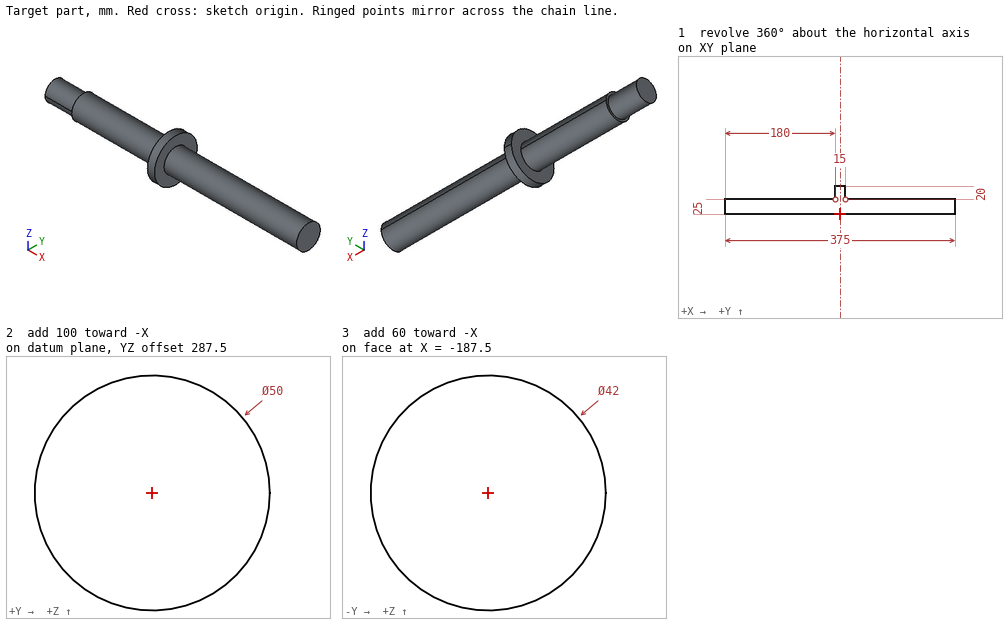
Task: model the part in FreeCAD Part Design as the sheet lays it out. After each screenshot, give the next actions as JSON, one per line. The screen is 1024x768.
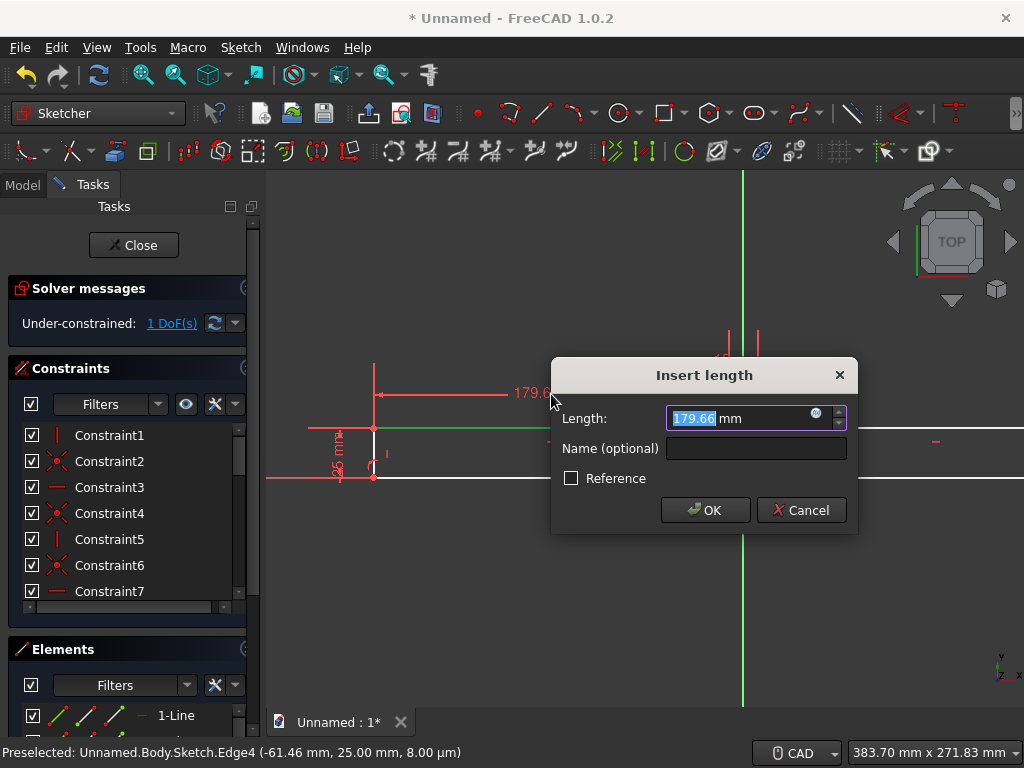
{"action": "type", "text": "180"}
{"action": "key", "text": "Return"}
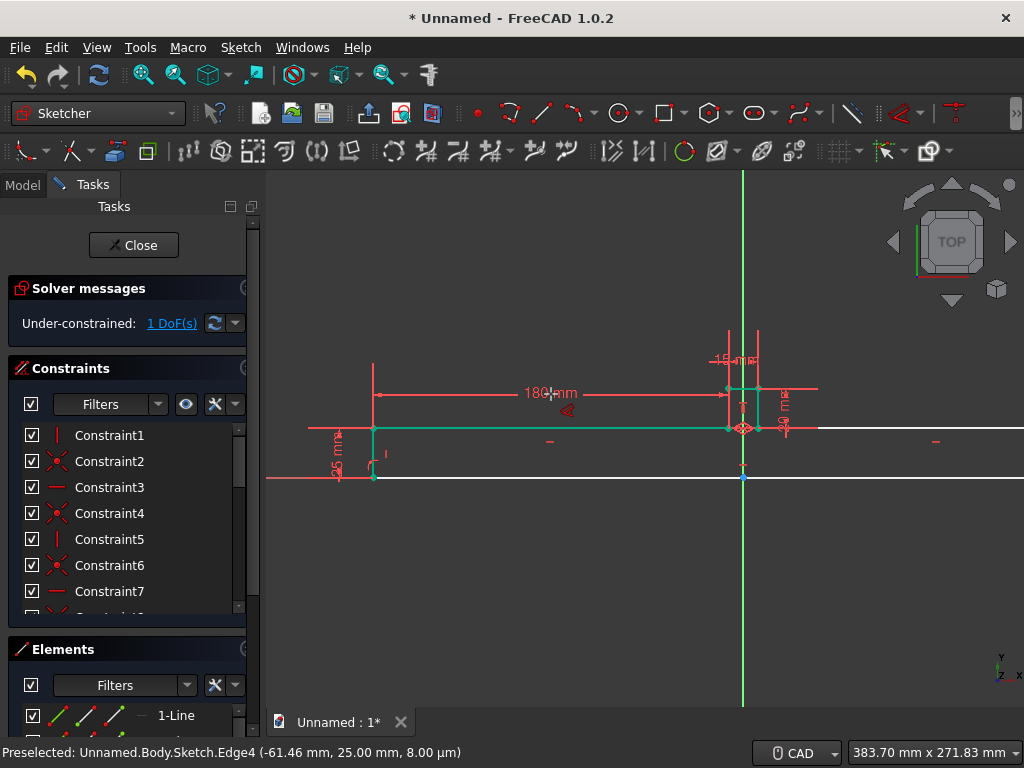
{"action": "left_click", "coordinate": [595, 478]}
{"action": "left_click", "coordinate": [616, 512]}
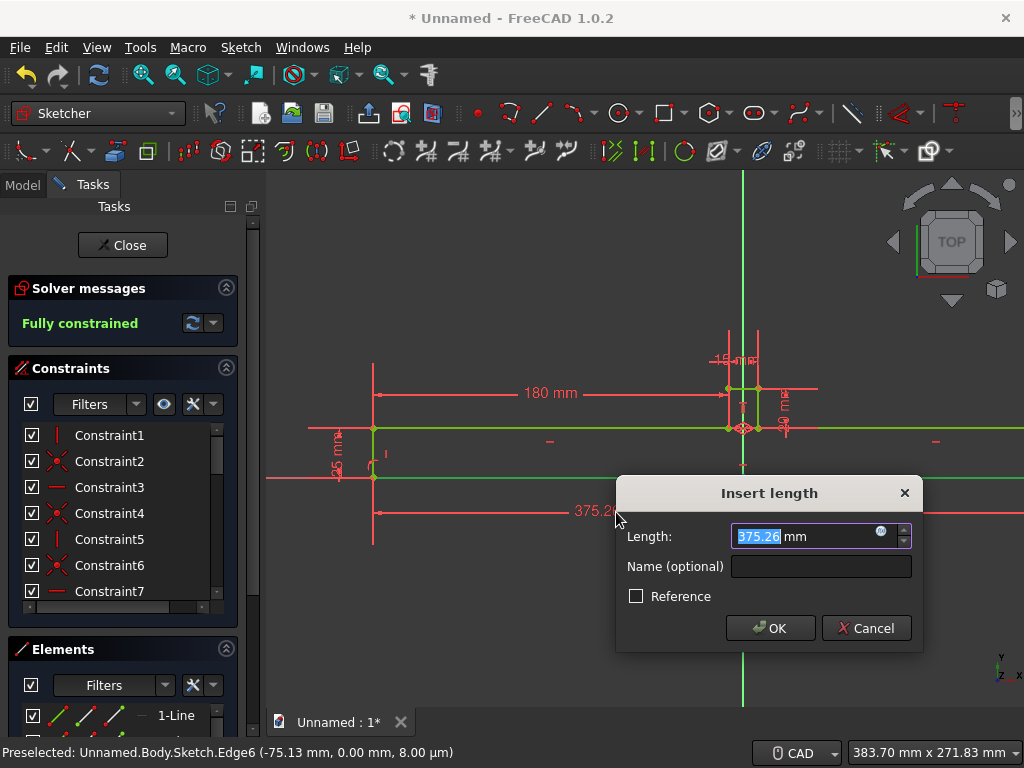
{"action": "type", "text": "375"}
{"action": "key", "text": "Return"}
{"action": "key", "text": "Escape"}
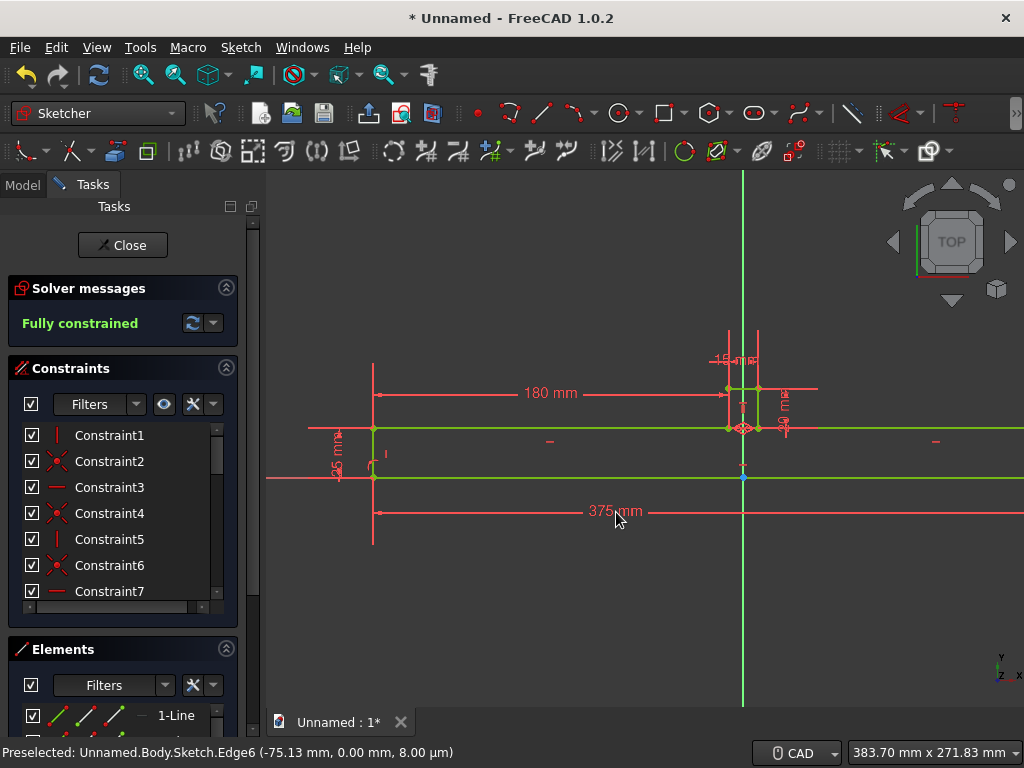
{"action": "left_click", "coordinate": [123, 245]}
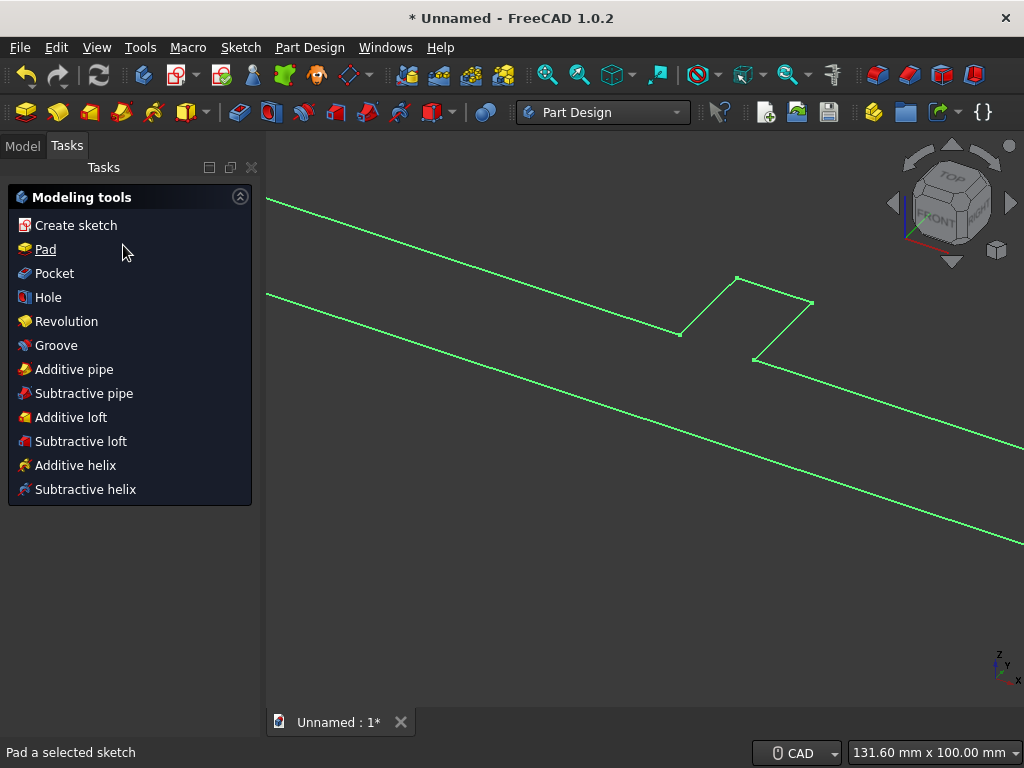
{"action": "left_click", "coordinate": [58, 112]}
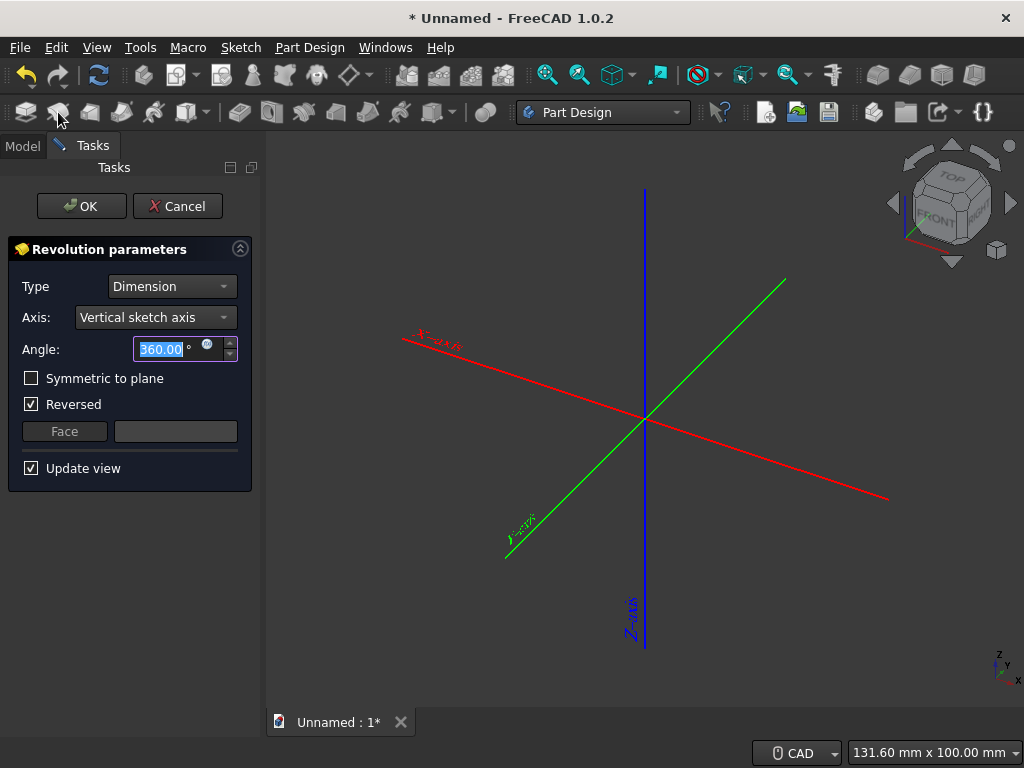
{"action": "left_click", "coordinate": [156, 318]}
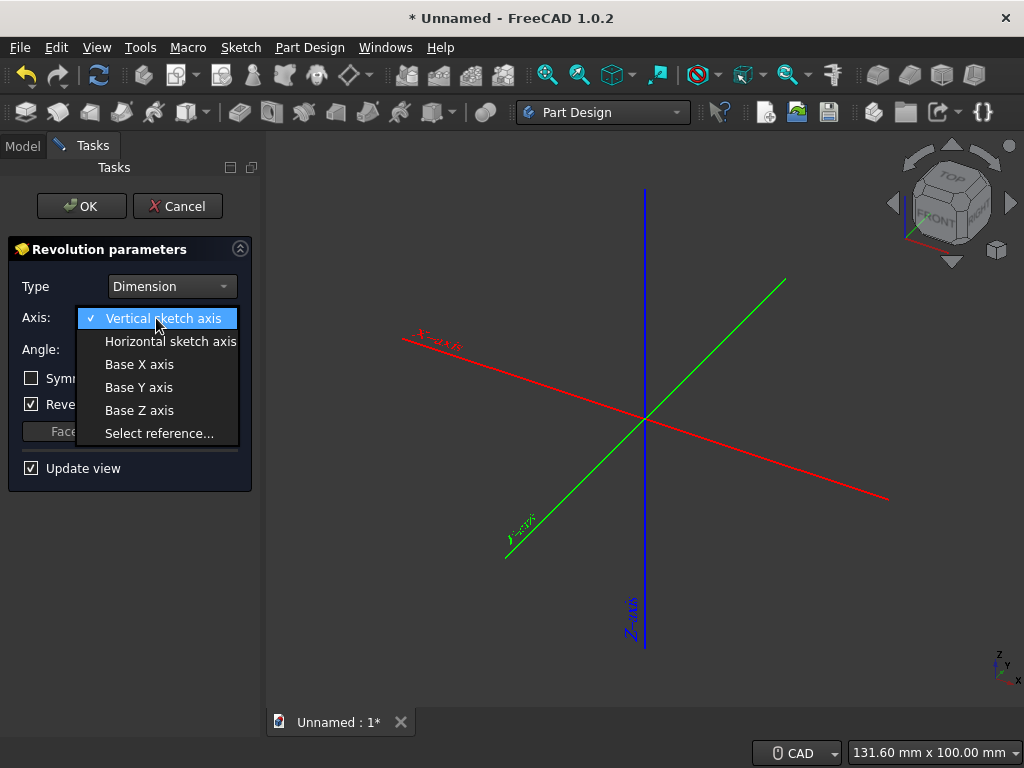
{"action": "left_click", "coordinate": [156, 342]}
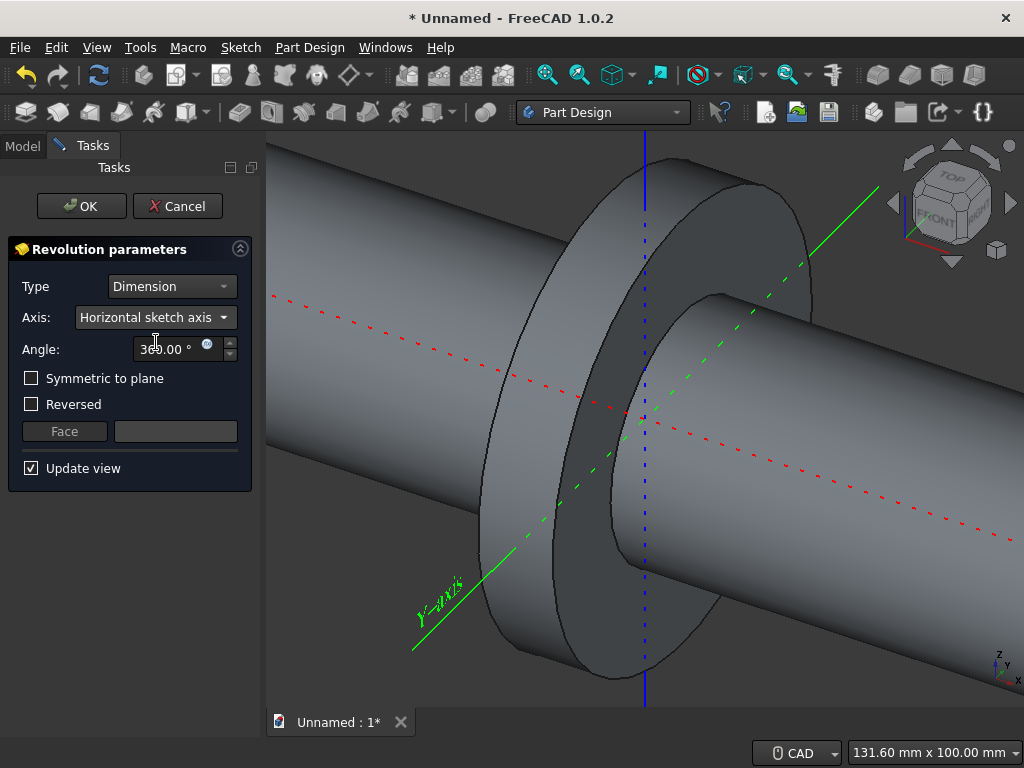
{"action": "left_click", "coordinate": [82, 206]}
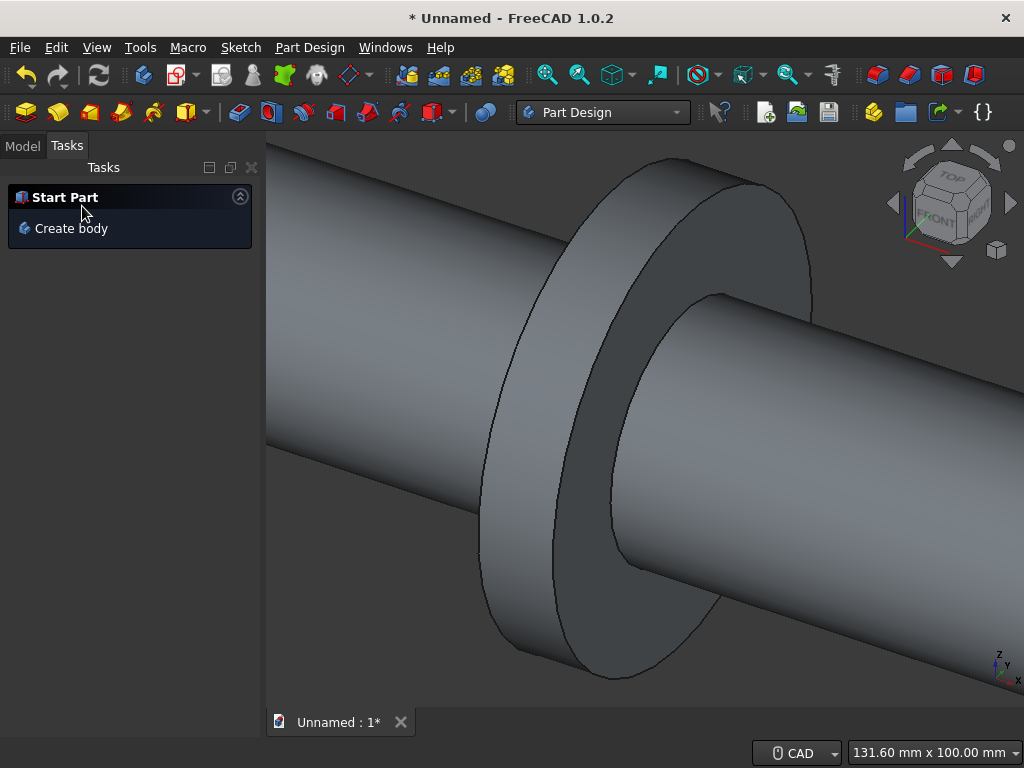
{"action": "key", "text": "v f"}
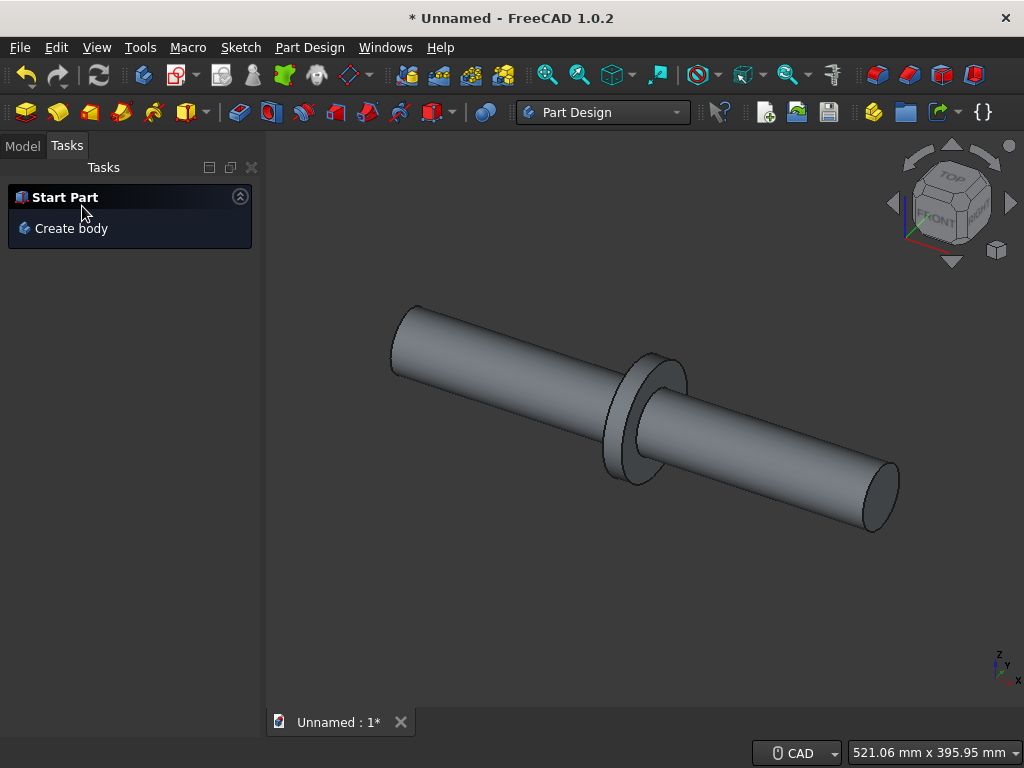
{"action": "left_click", "coordinate": [23, 145]}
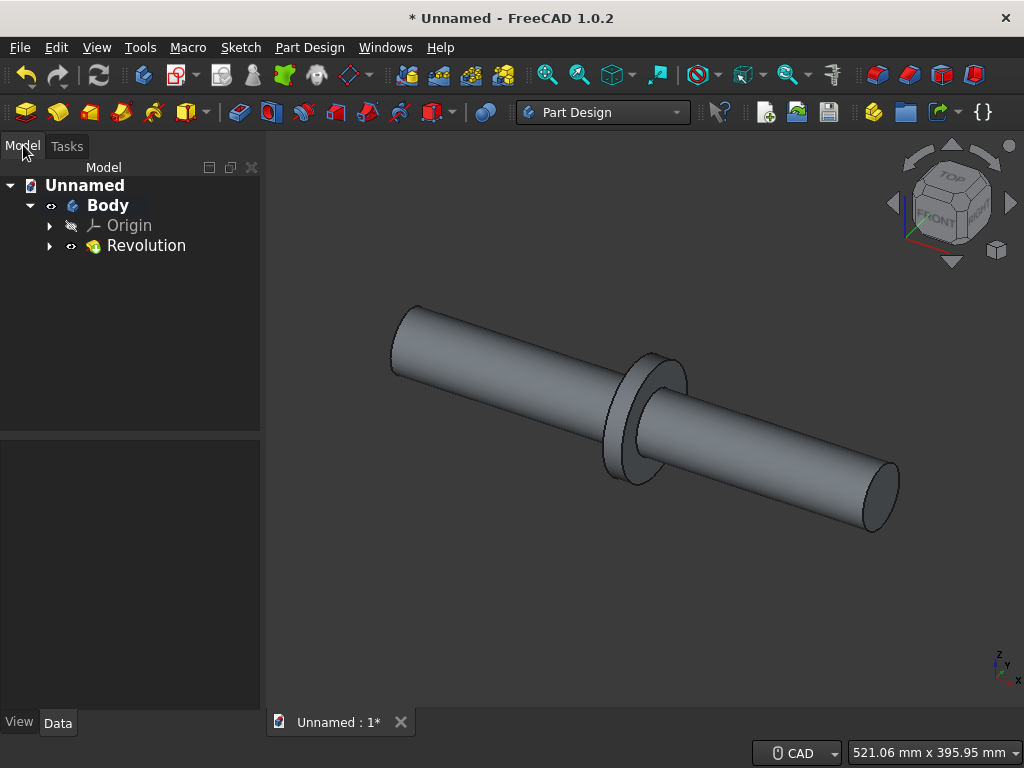
{"action": "left_click", "coordinate": [50, 226]}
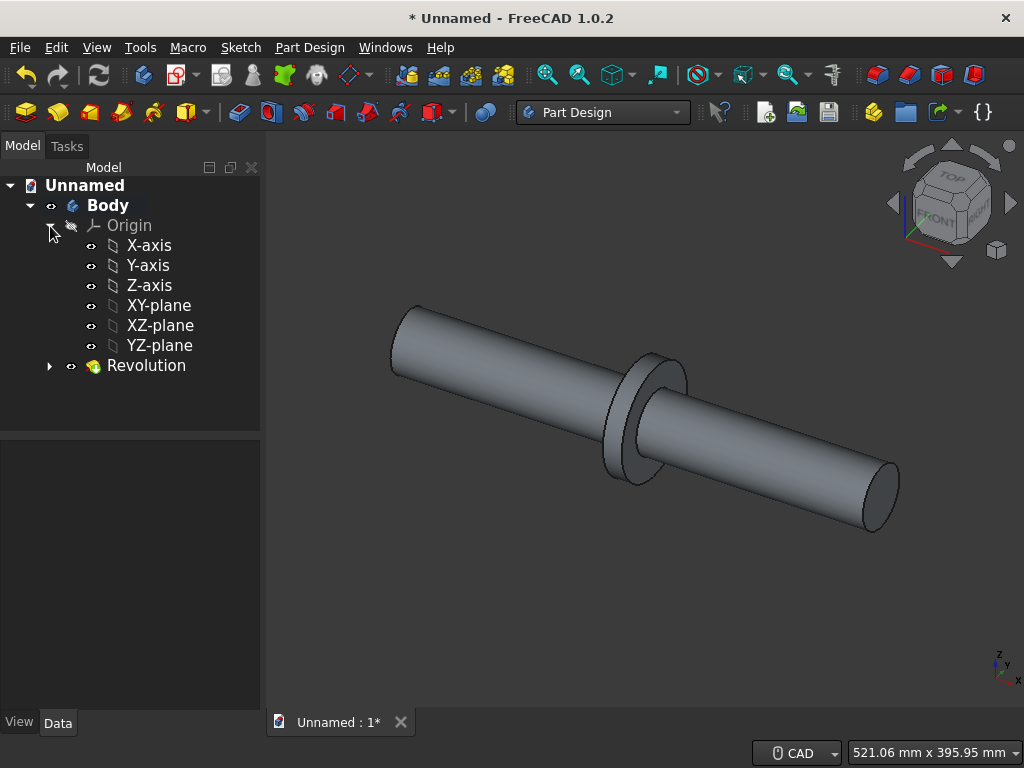
{"action": "left_click", "coordinate": [136, 346]}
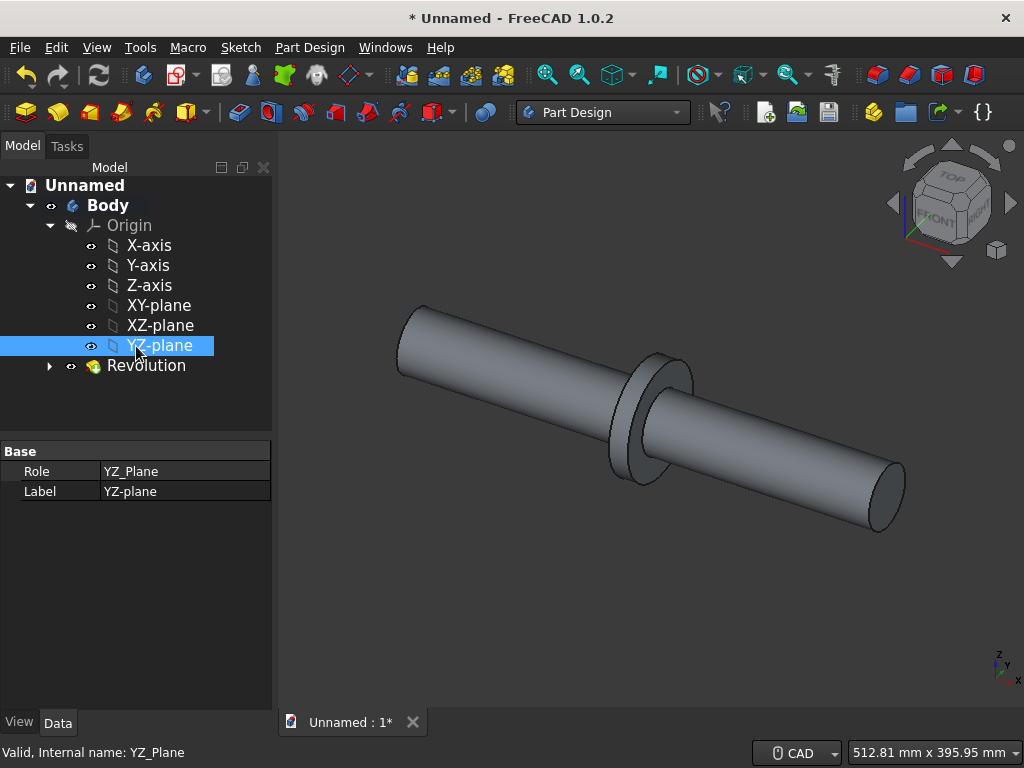
{"action": "left_click", "coordinate": [350, 76]}